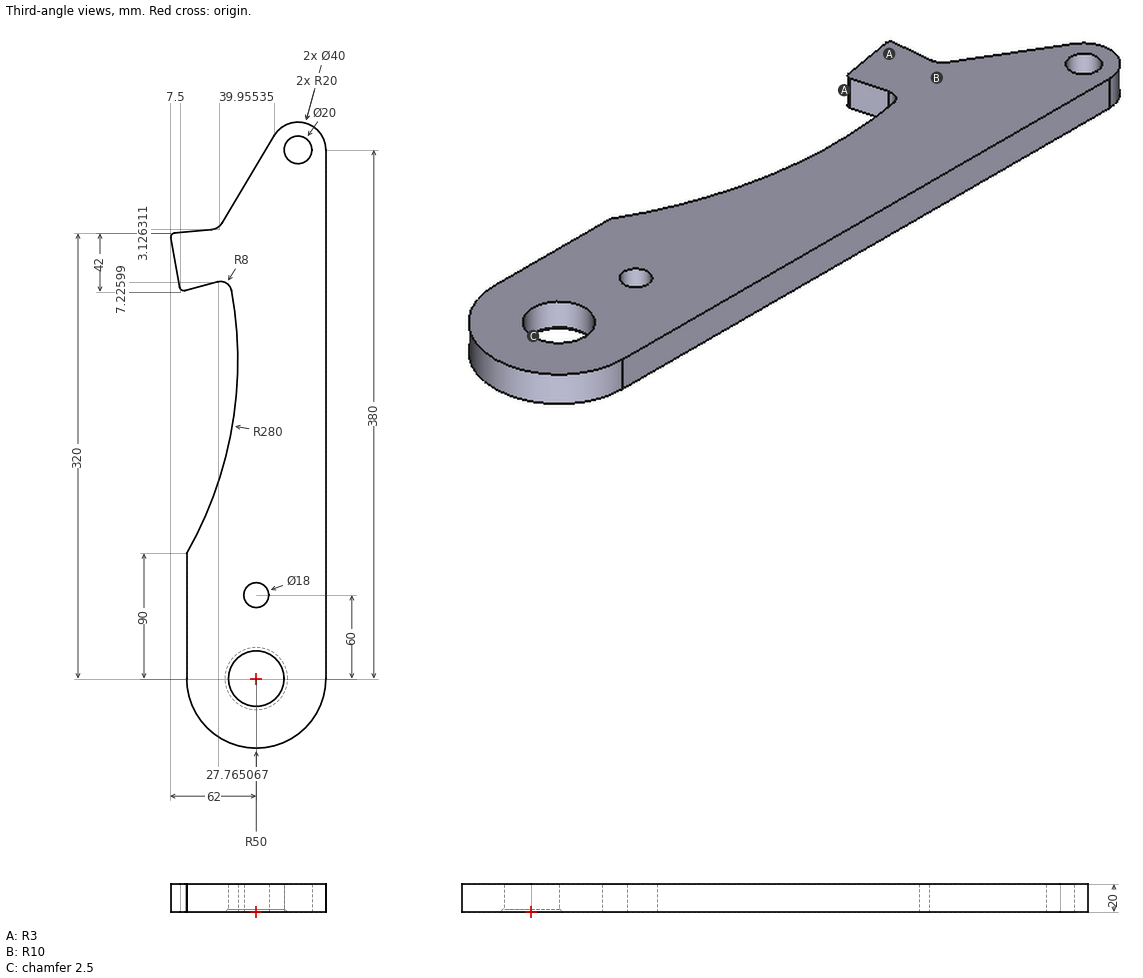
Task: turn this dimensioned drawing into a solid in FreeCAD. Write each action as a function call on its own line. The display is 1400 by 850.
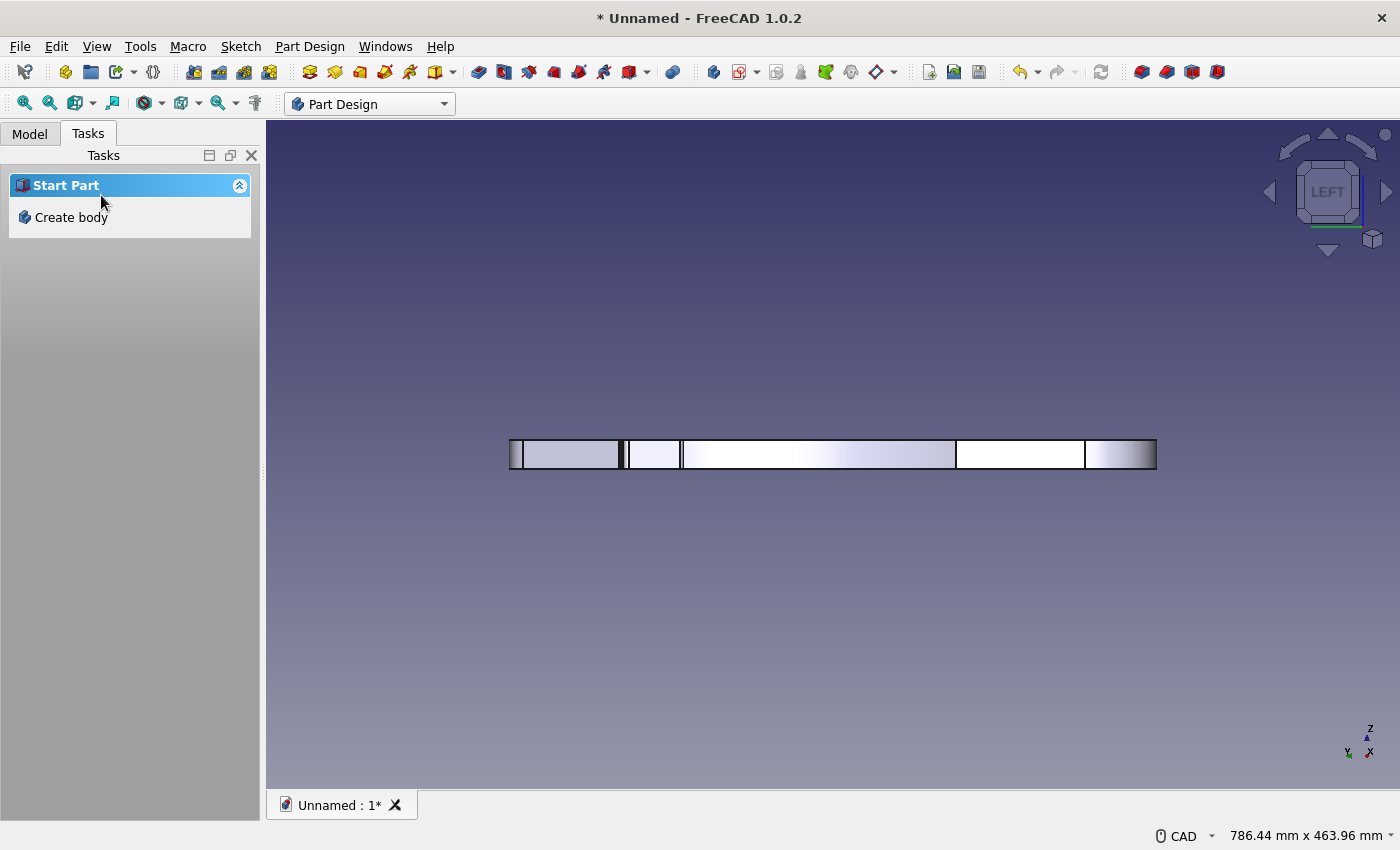
key(v)
key(3)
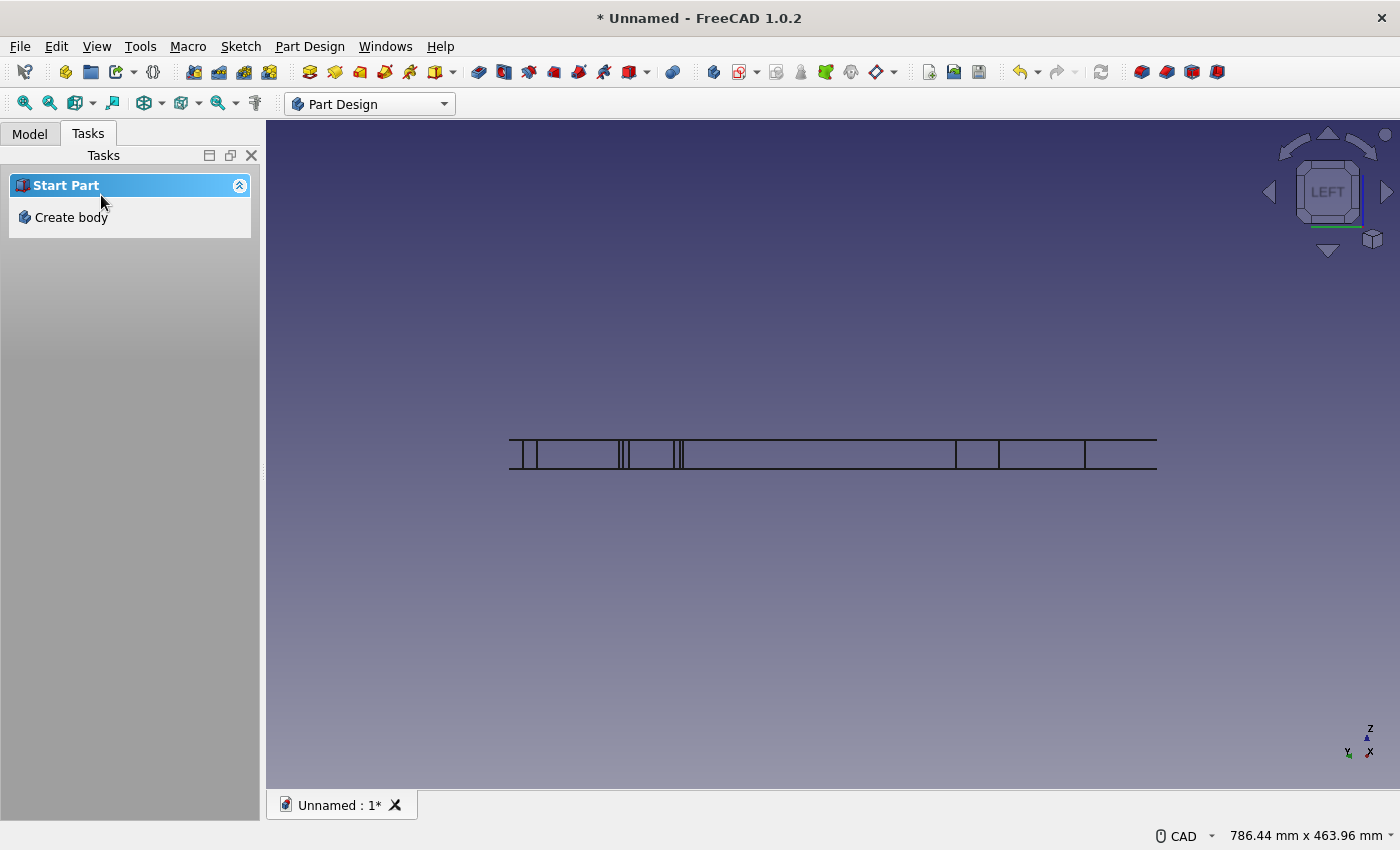
key(0)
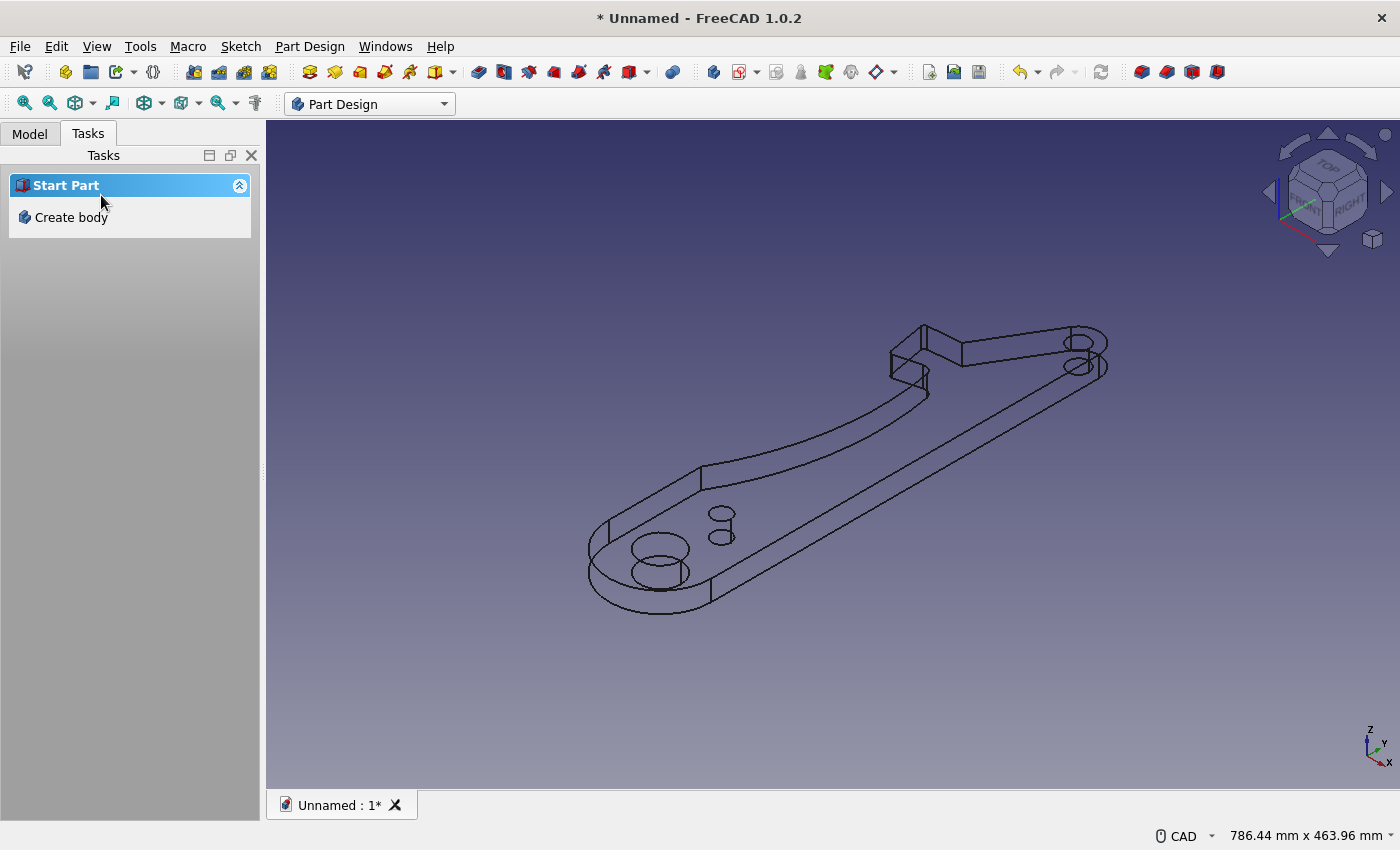
click(962, 354)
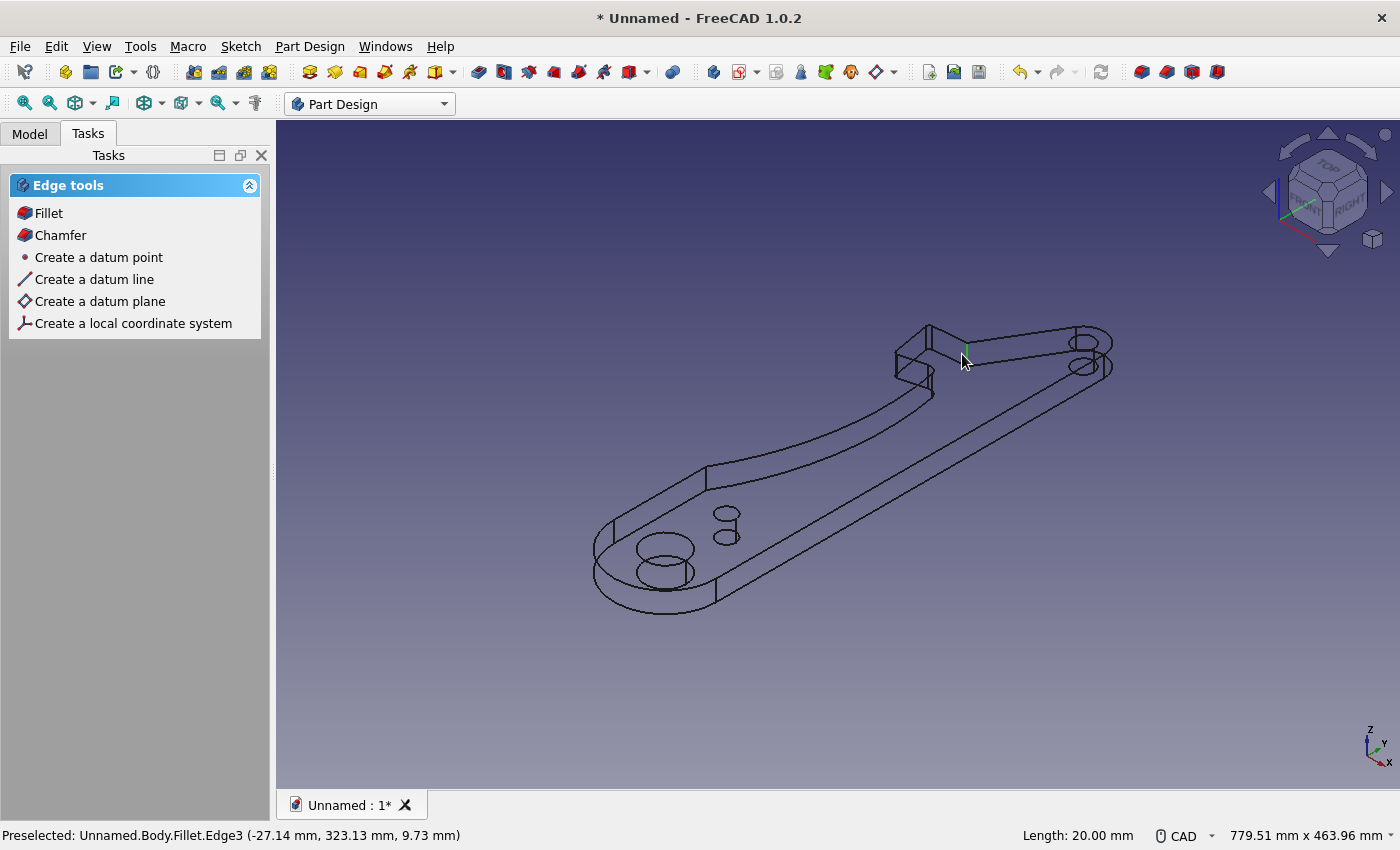
key(v)
key(1)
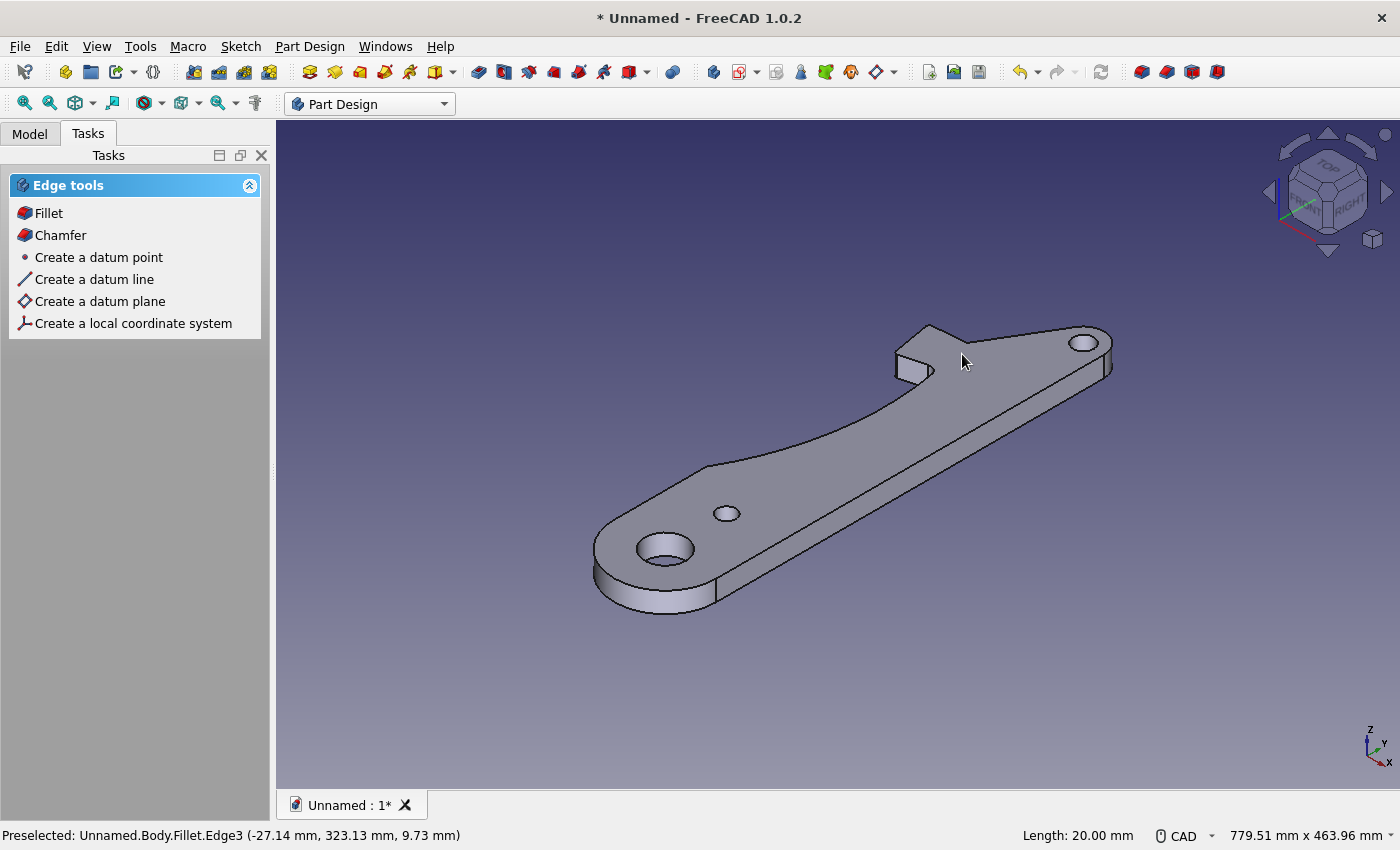
click(1142, 72)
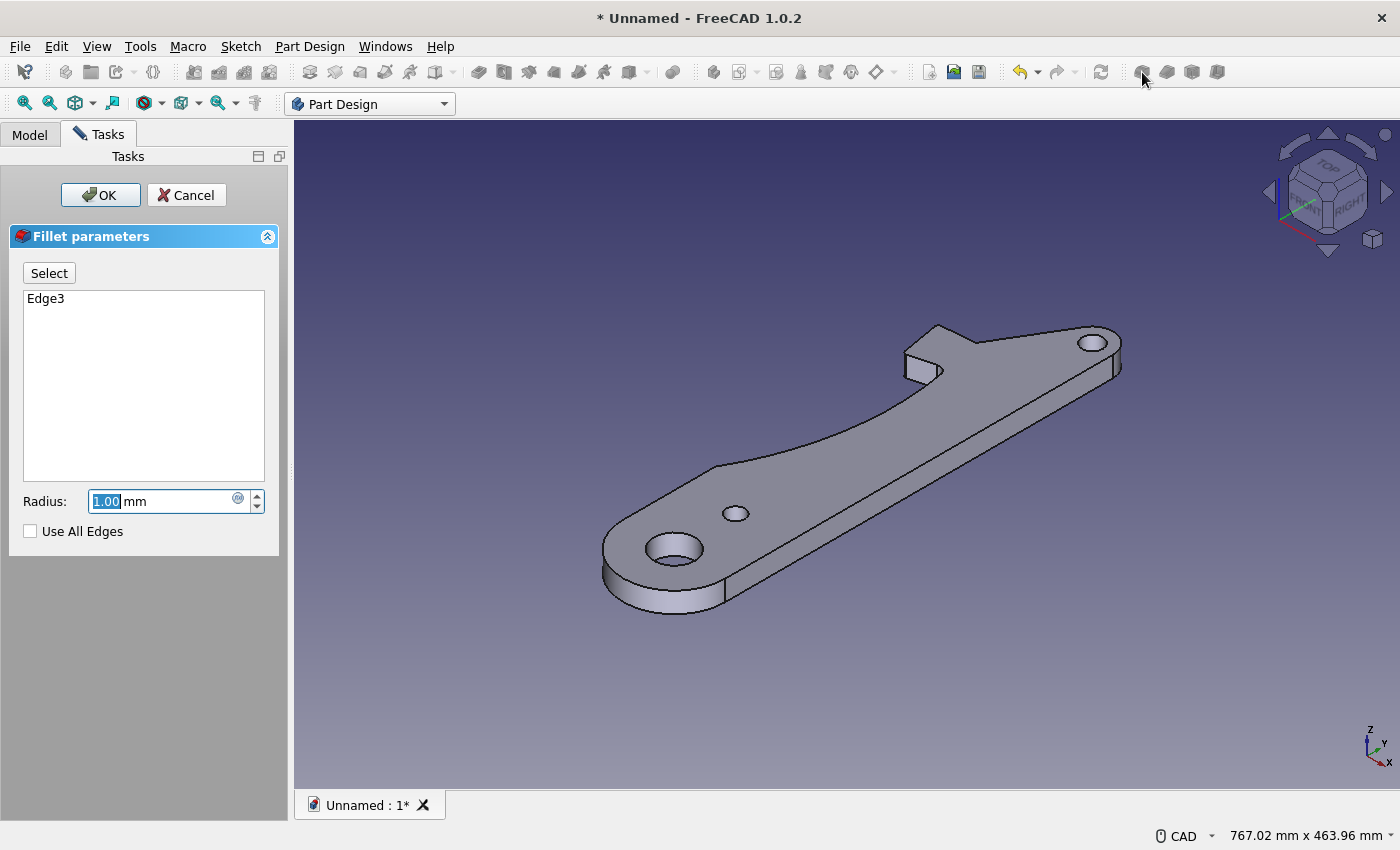
text(10)
key(Tab)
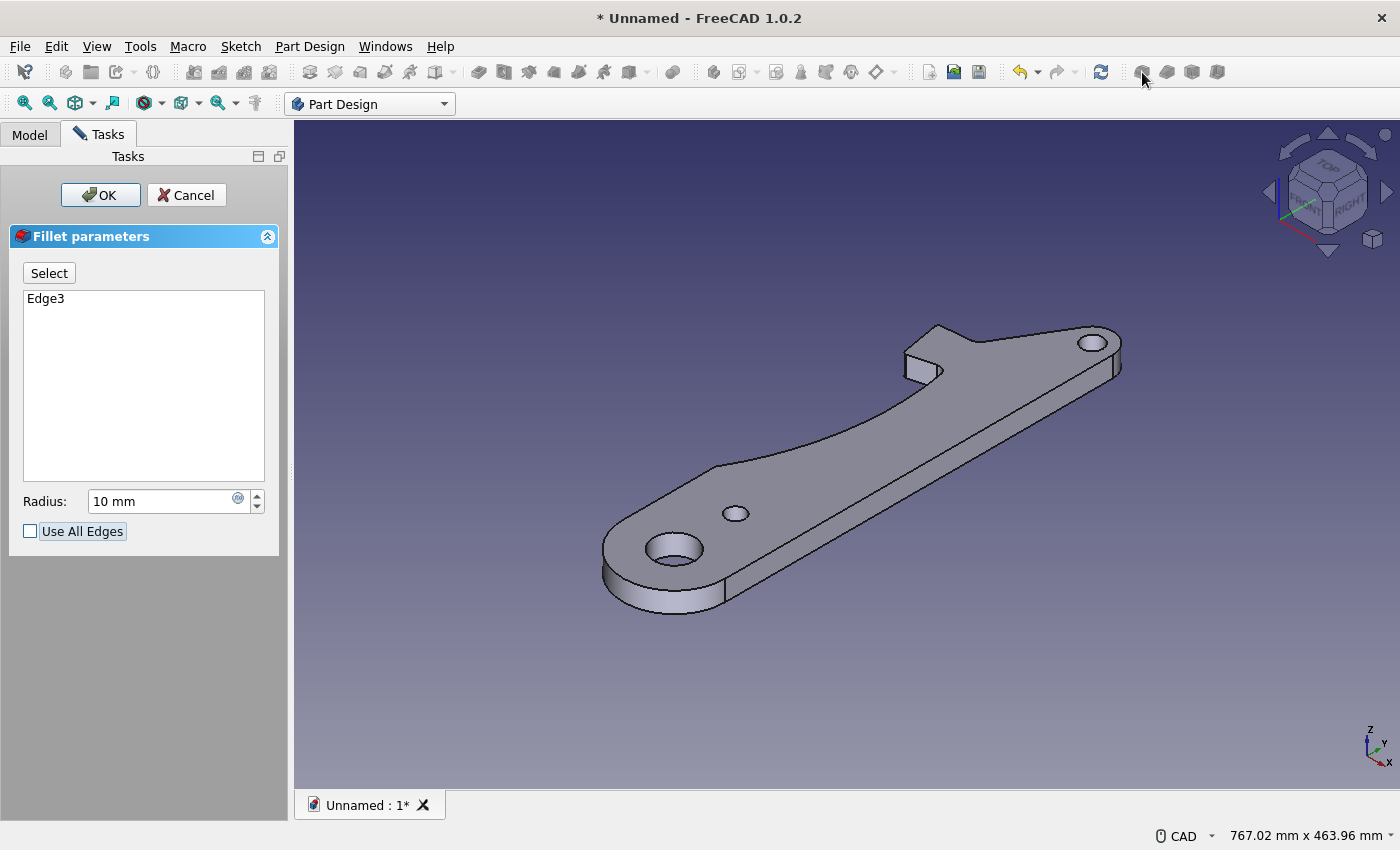
click(101, 195)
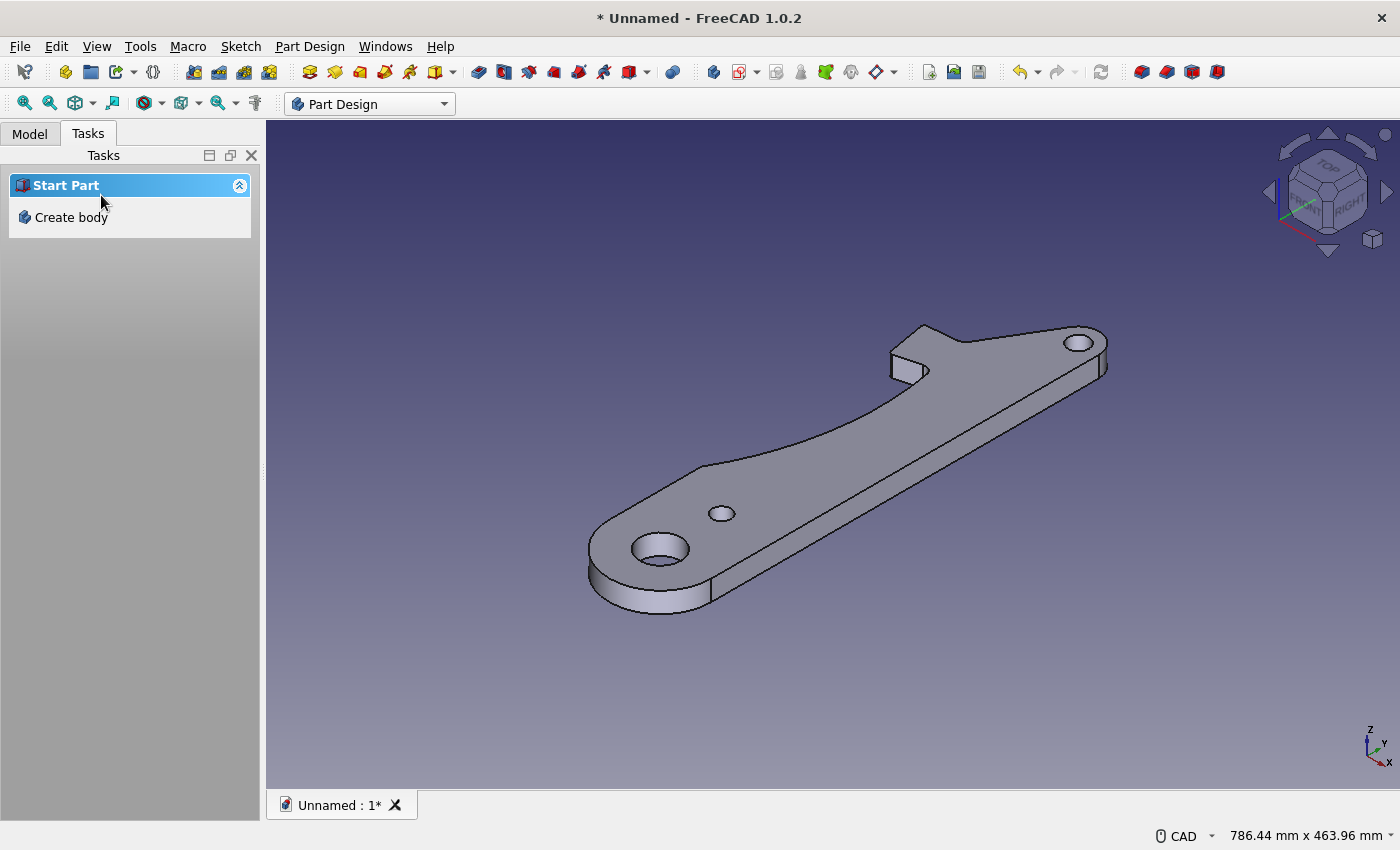
key(2)